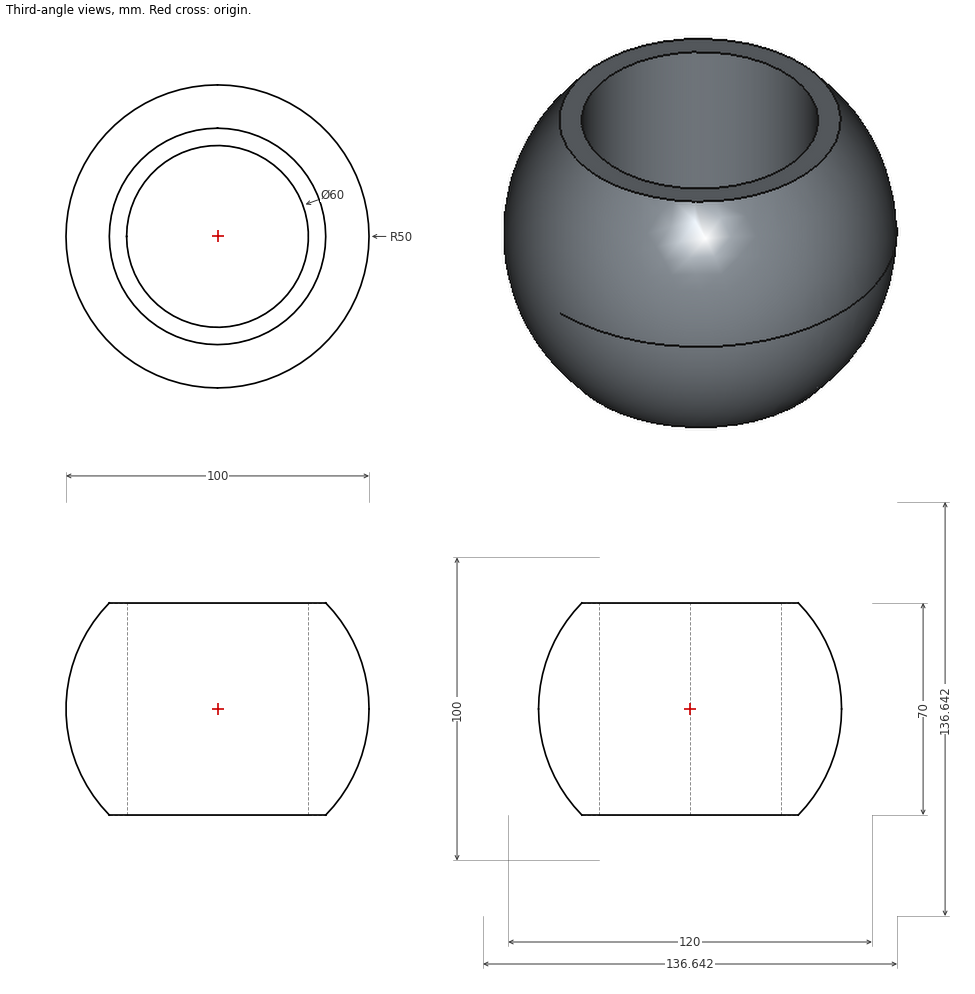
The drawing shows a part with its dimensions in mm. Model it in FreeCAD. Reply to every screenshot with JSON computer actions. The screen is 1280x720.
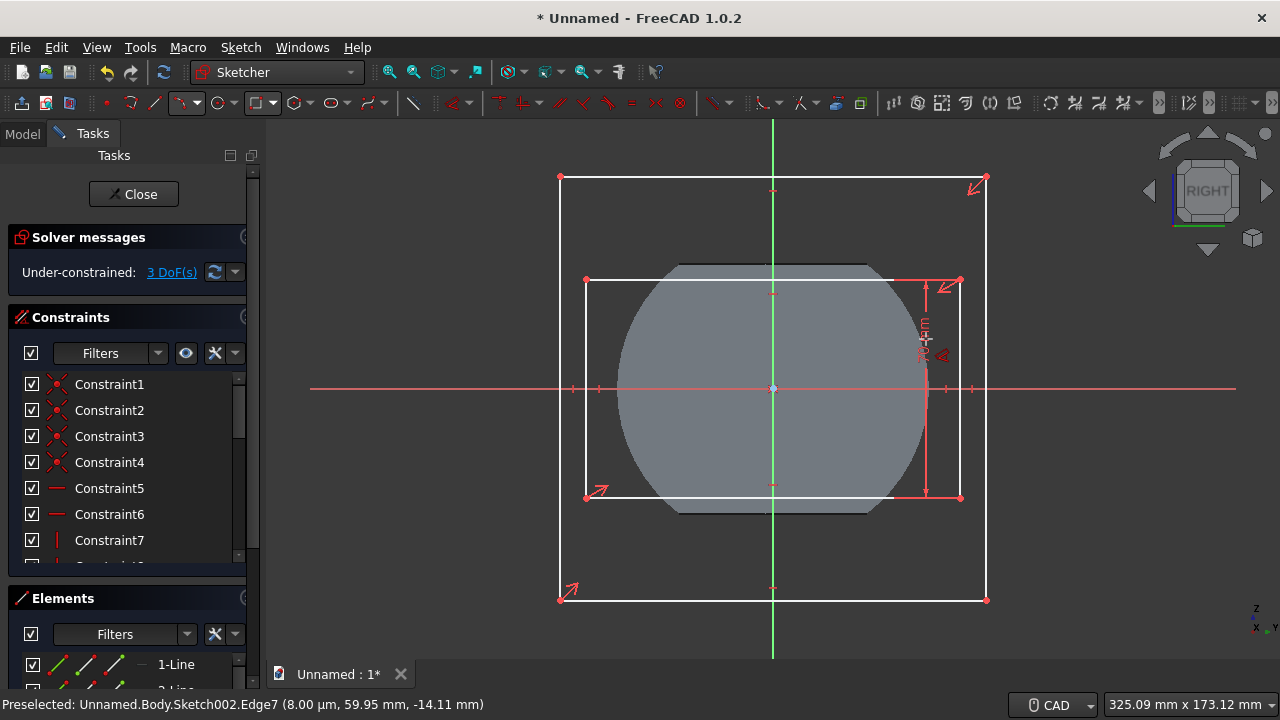
{"action": "left_click", "coordinate": [698, 498]}
{"action": "left_click", "coordinate": [687, 532]}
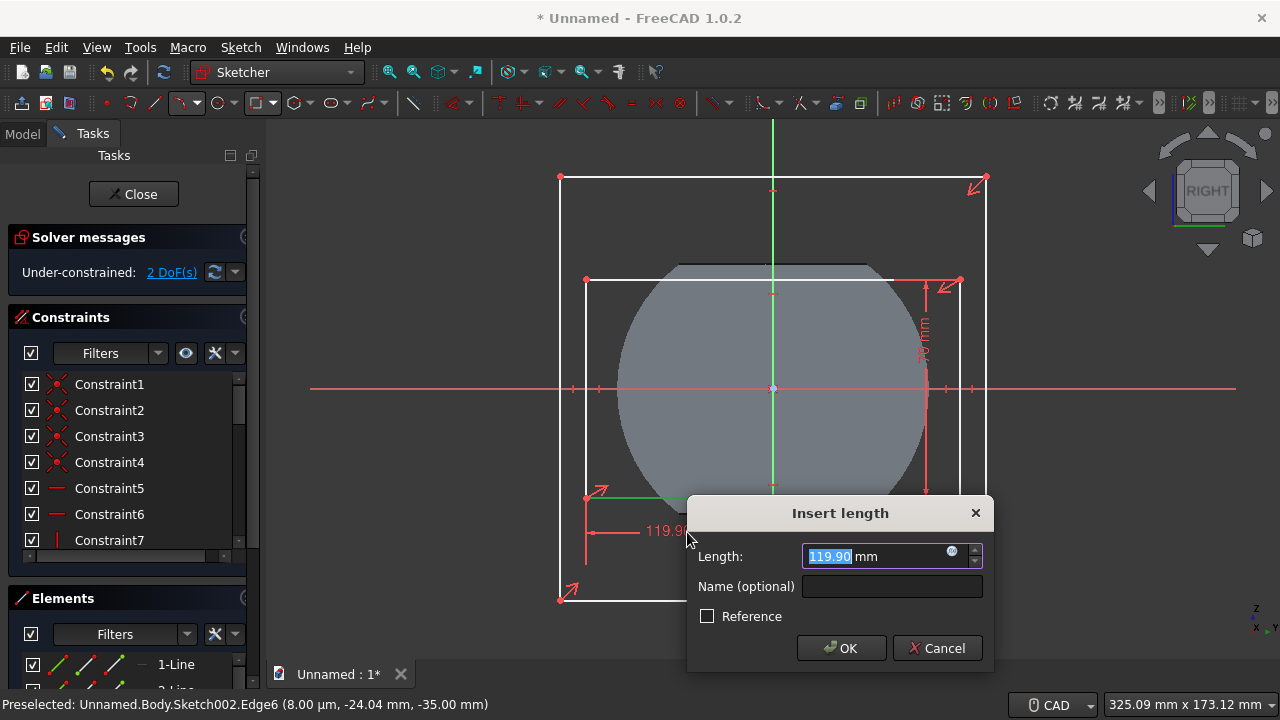
{"action": "type", "text": "120"}
{"action": "key", "text": "Return"}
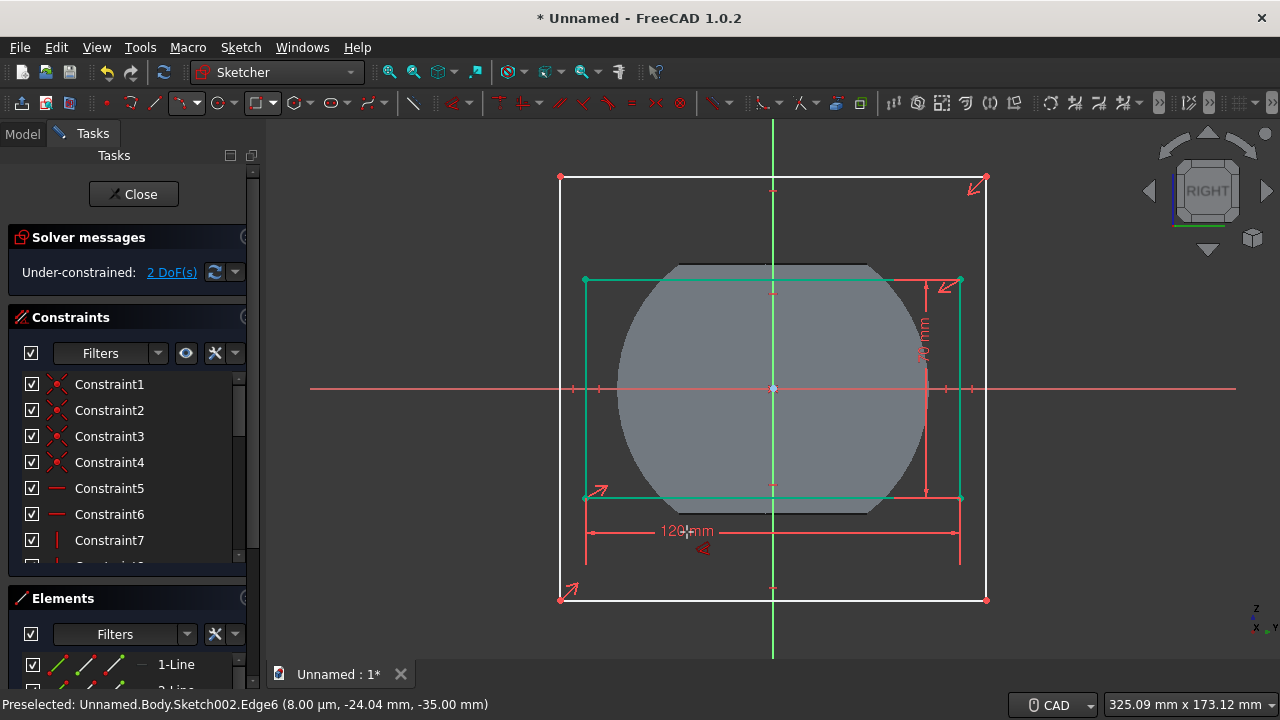
{"action": "left_click", "coordinate": [688, 601]}
{"action": "left_click", "coordinate": [675, 567]}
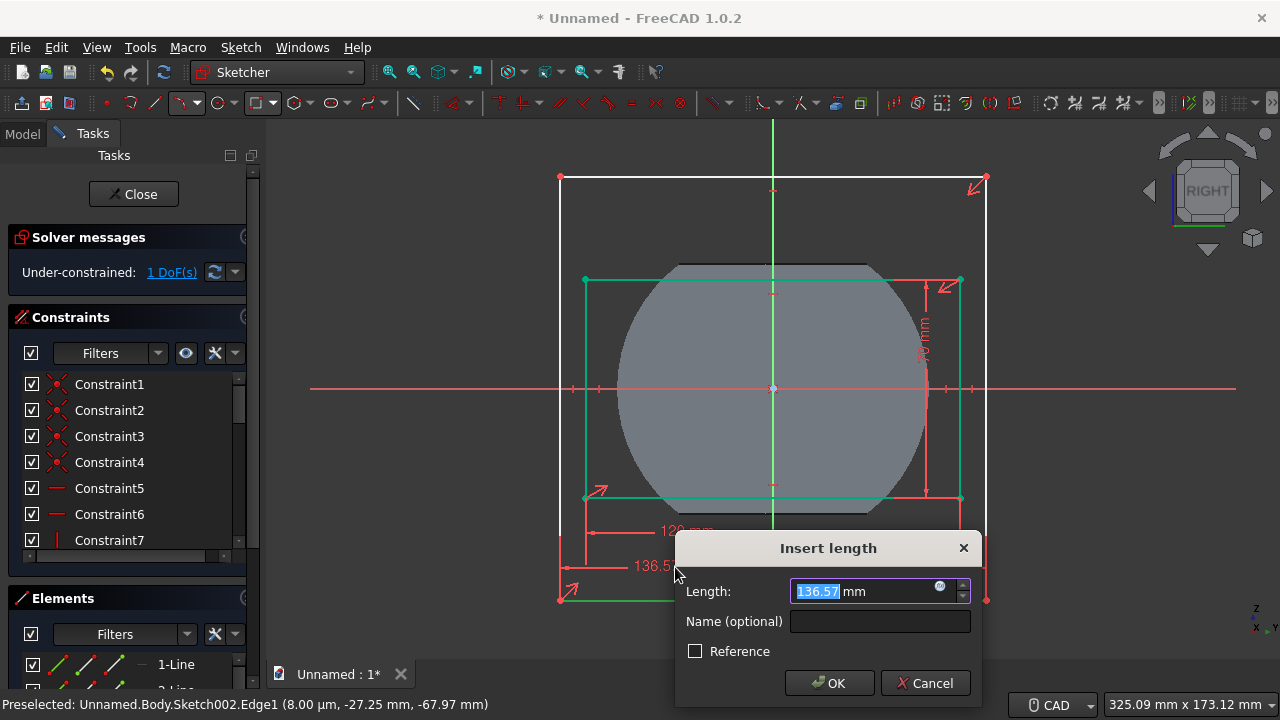
{"action": "type", "text": "136.642"}
{"action": "key", "text": "Return"}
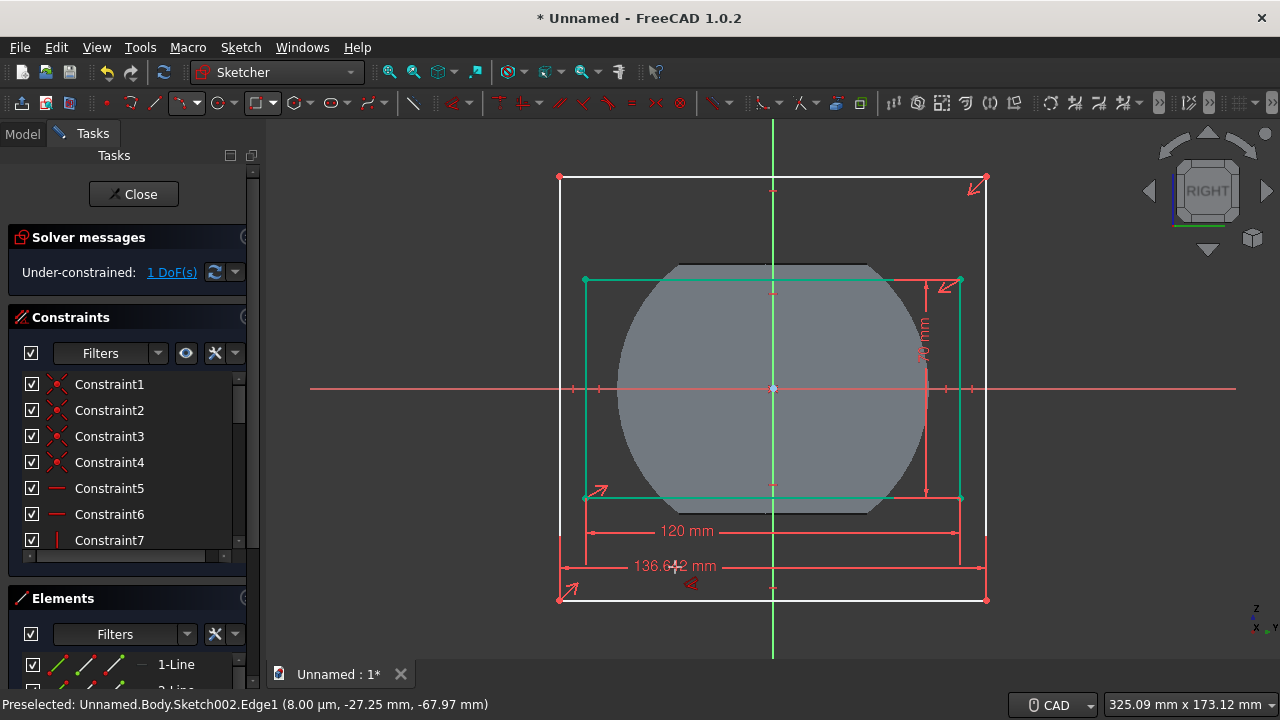
{"action": "left_click", "coordinate": [986, 474]}
{"action": "left_click", "coordinate": [1020, 291]}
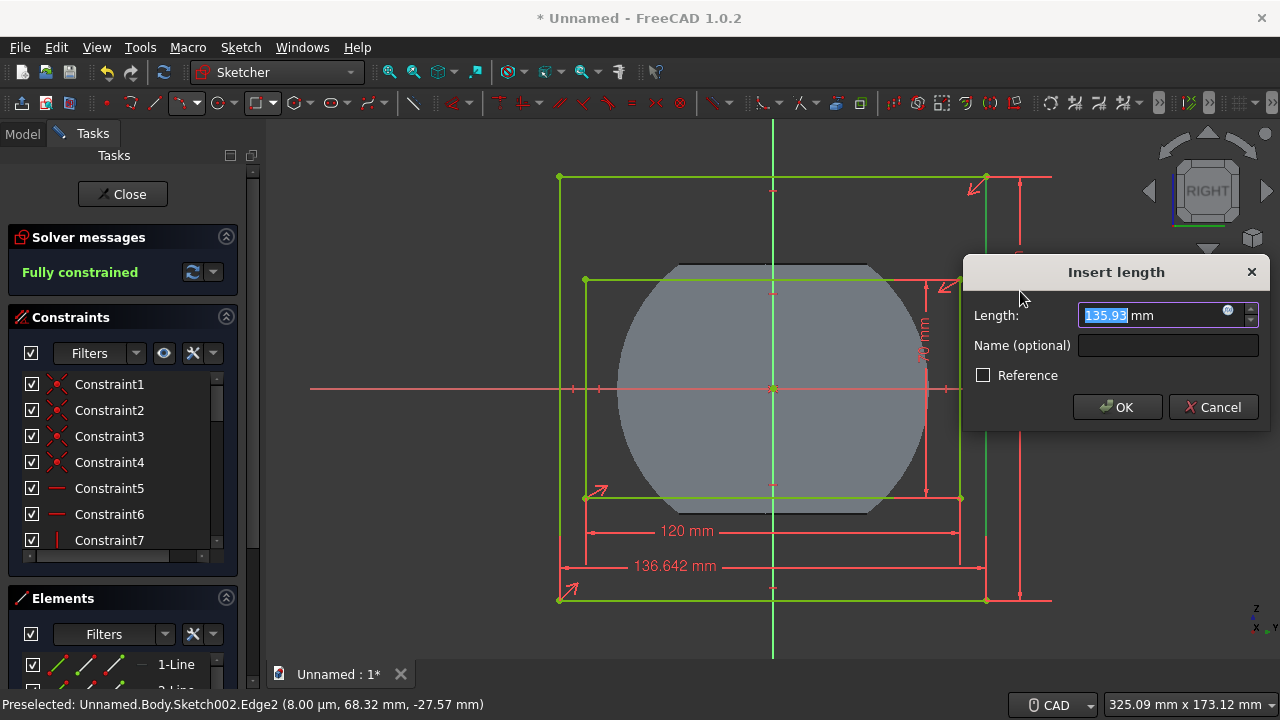
{"action": "type", "text": "136.642"}
{"action": "key", "text": "Return"}
{"action": "key", "text": "Escape"}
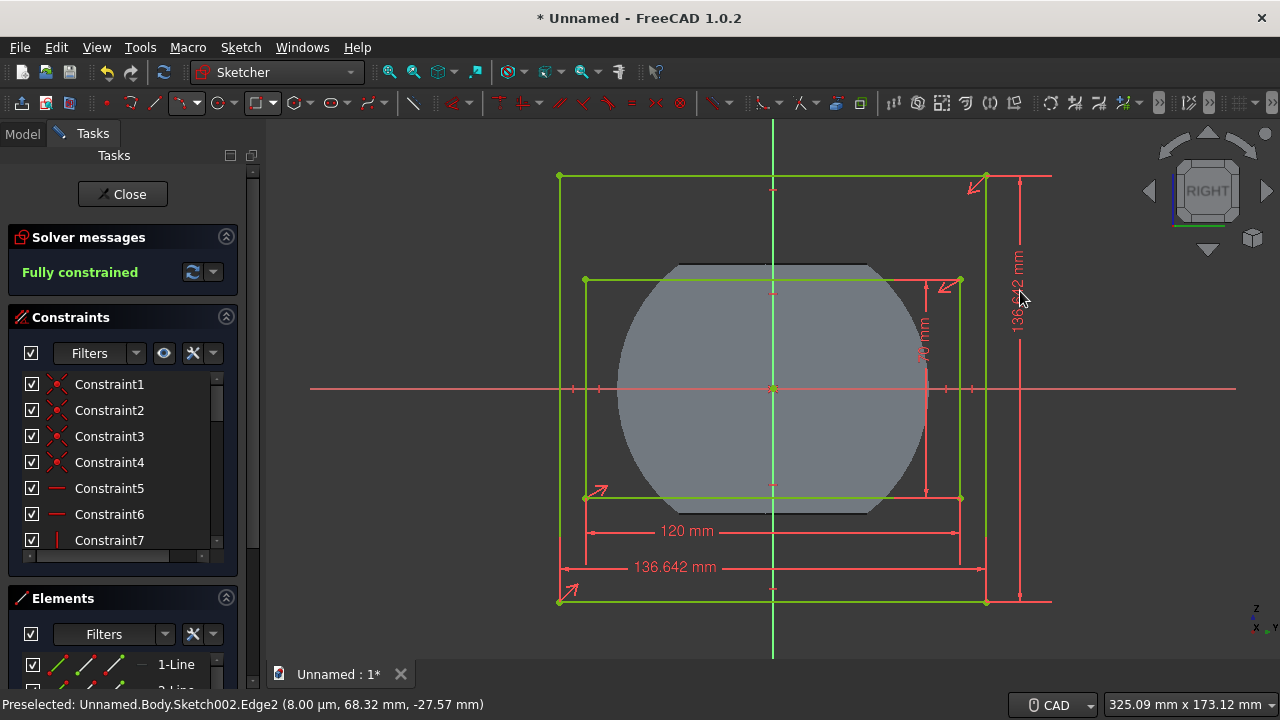
{"action": "left_click", "coordinate": [123, 194]}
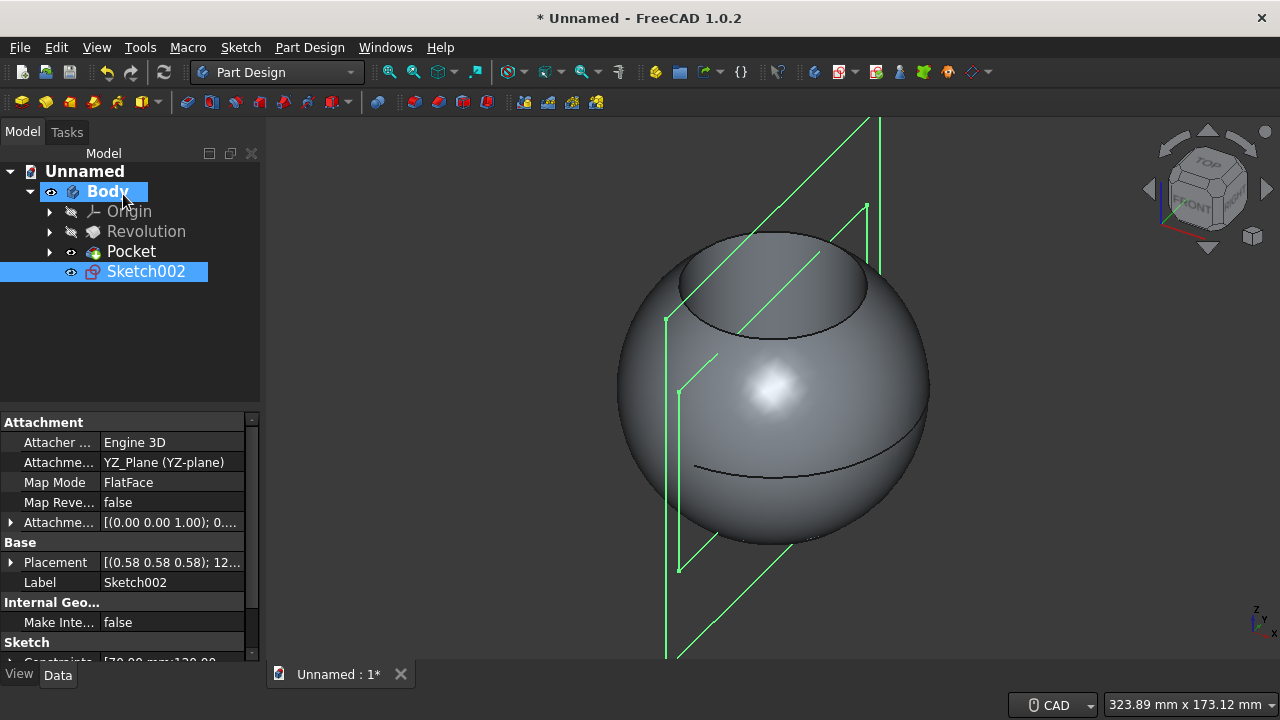
{"action": "left_click", "coordinate": [188, 102]}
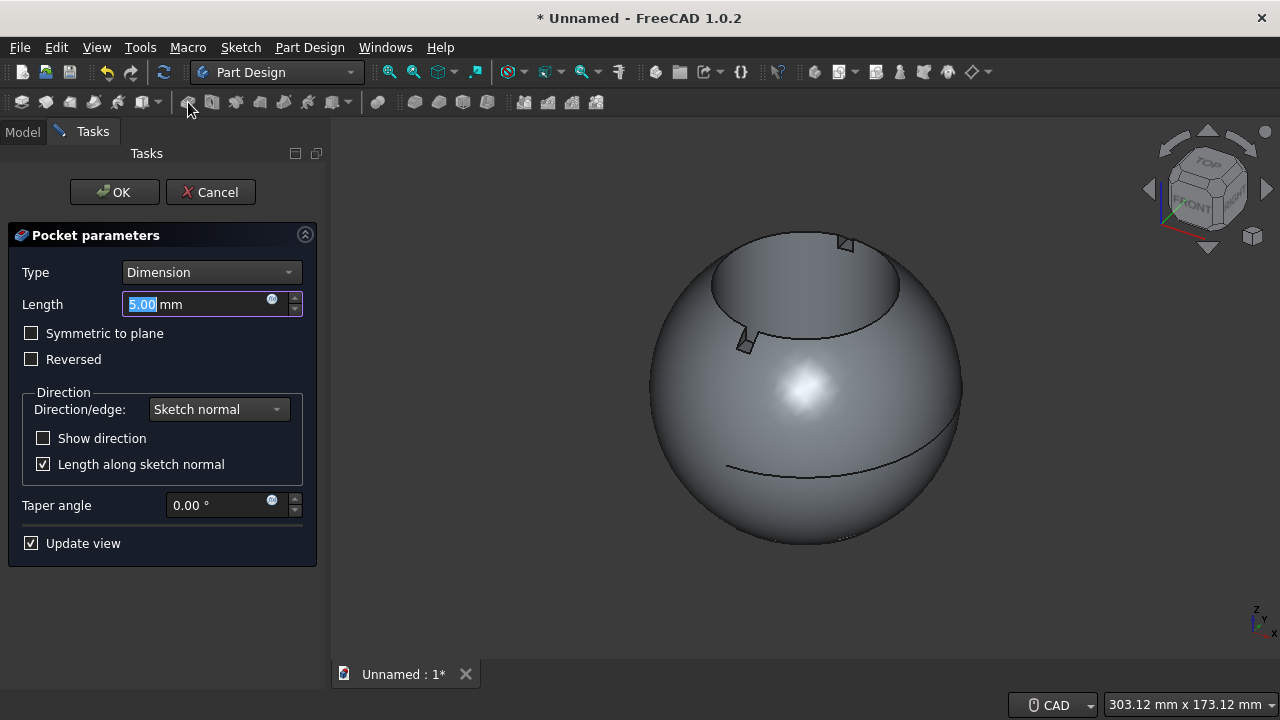
{"action": "type", "text": "100"}
{"action": "key", "text": "Tab"}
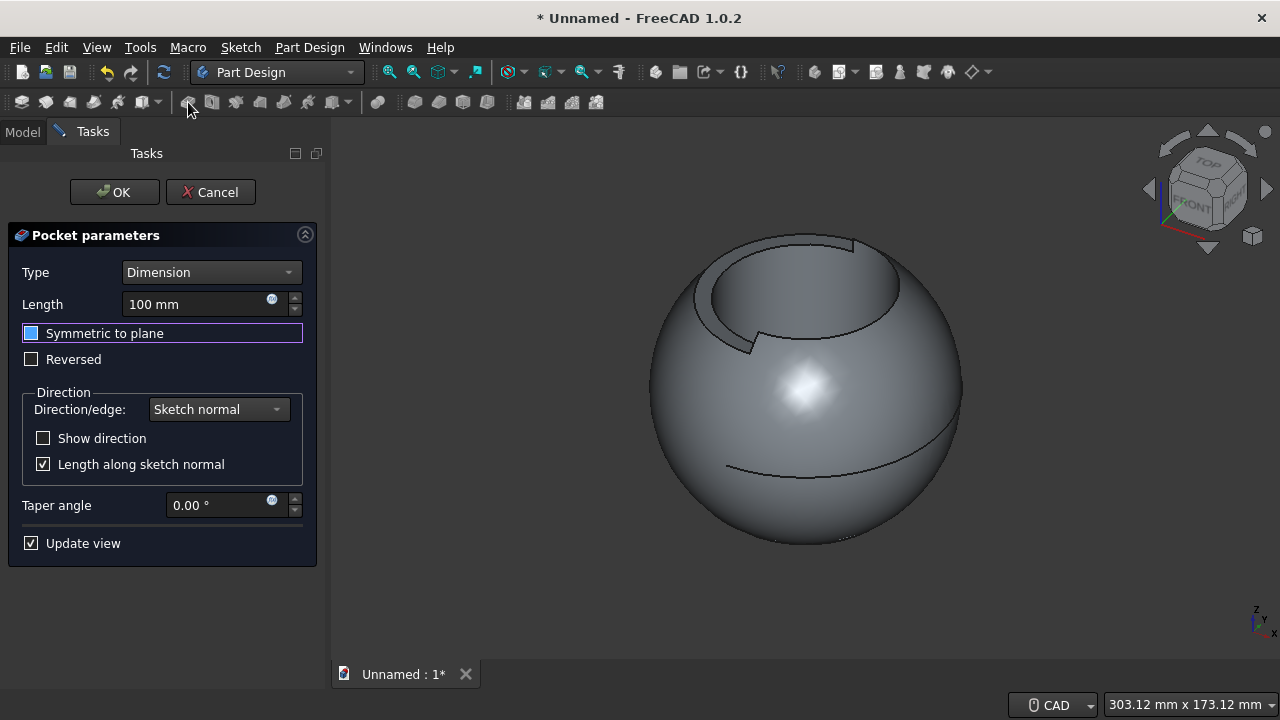
{"action": "left_click", "coordinate": [30, 333]}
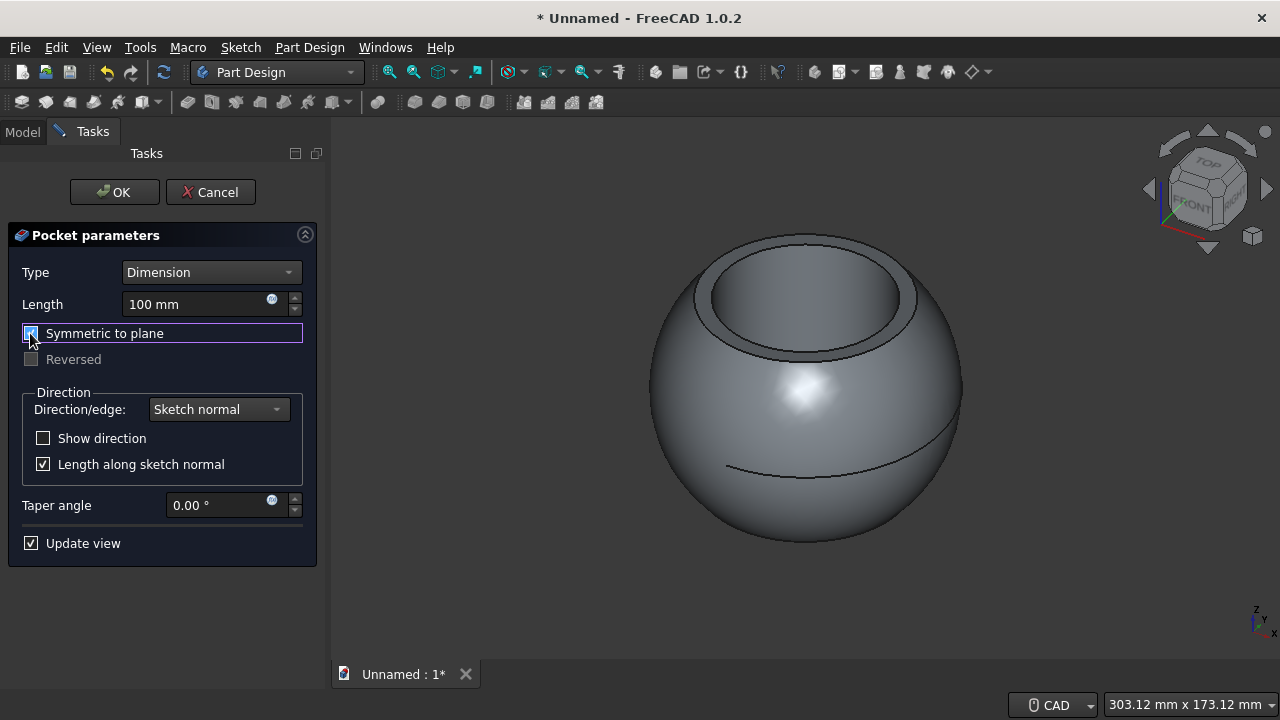
{"action": "left_click", "coordinate": [115, 192]}